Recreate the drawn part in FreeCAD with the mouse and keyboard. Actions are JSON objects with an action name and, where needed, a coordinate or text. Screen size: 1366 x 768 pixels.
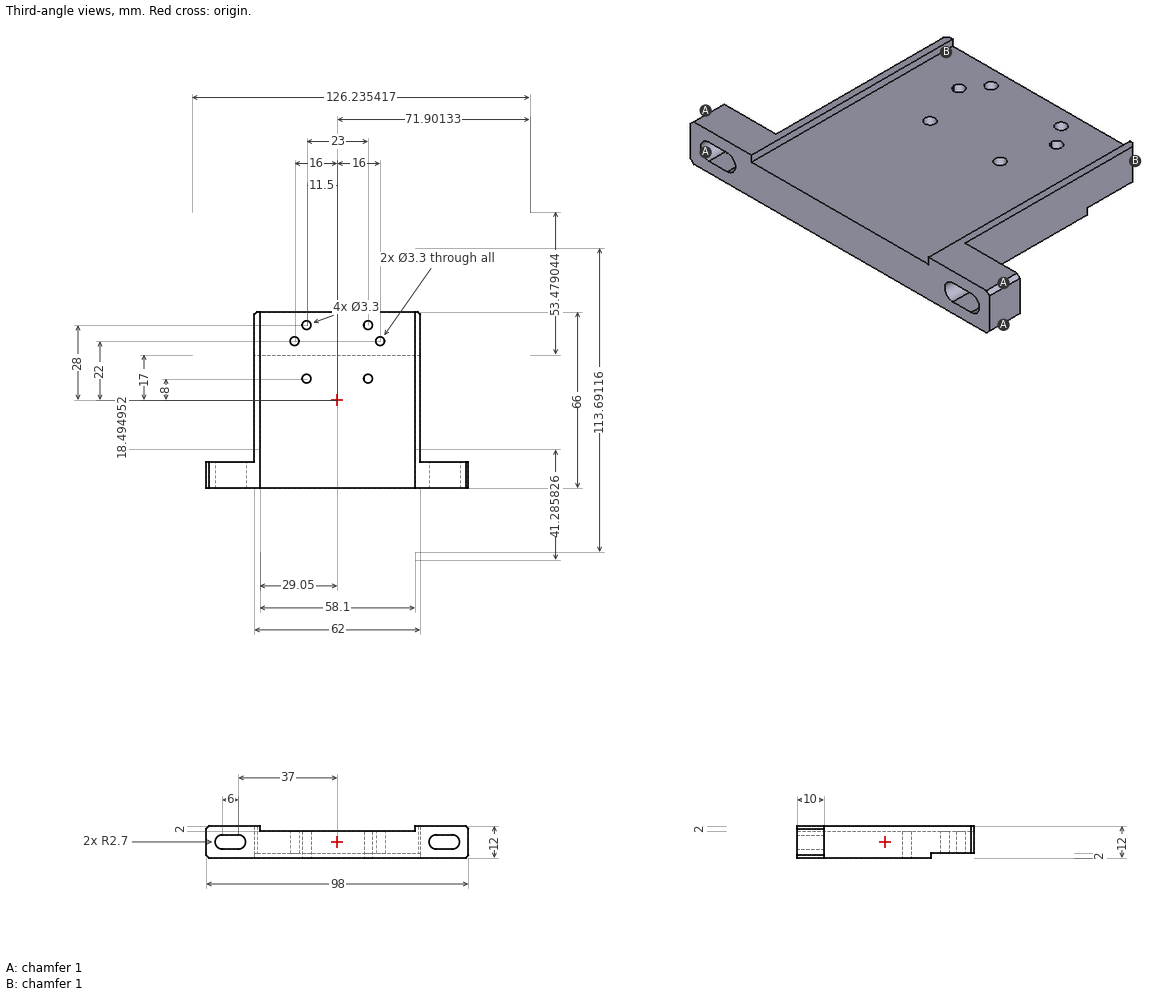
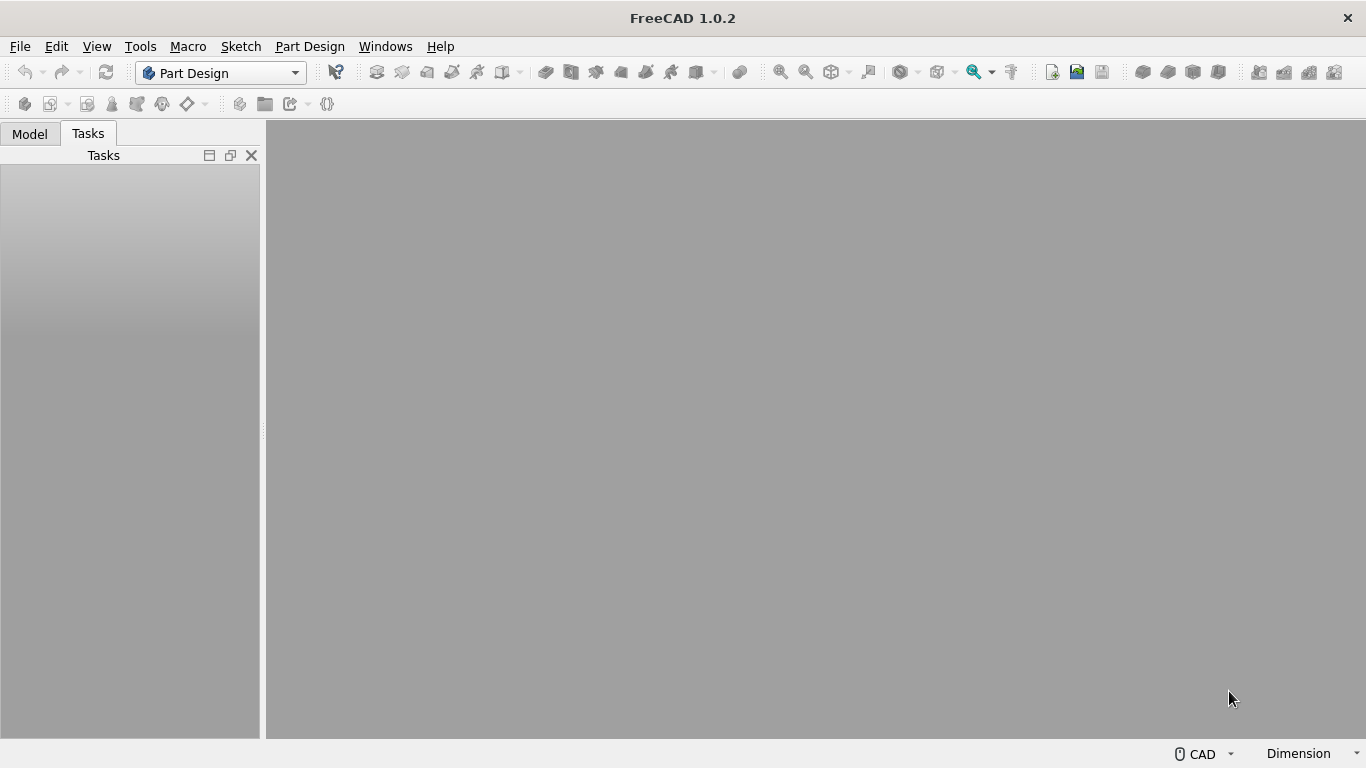
{"action": "left_click", "coordinate": [1052, 72]}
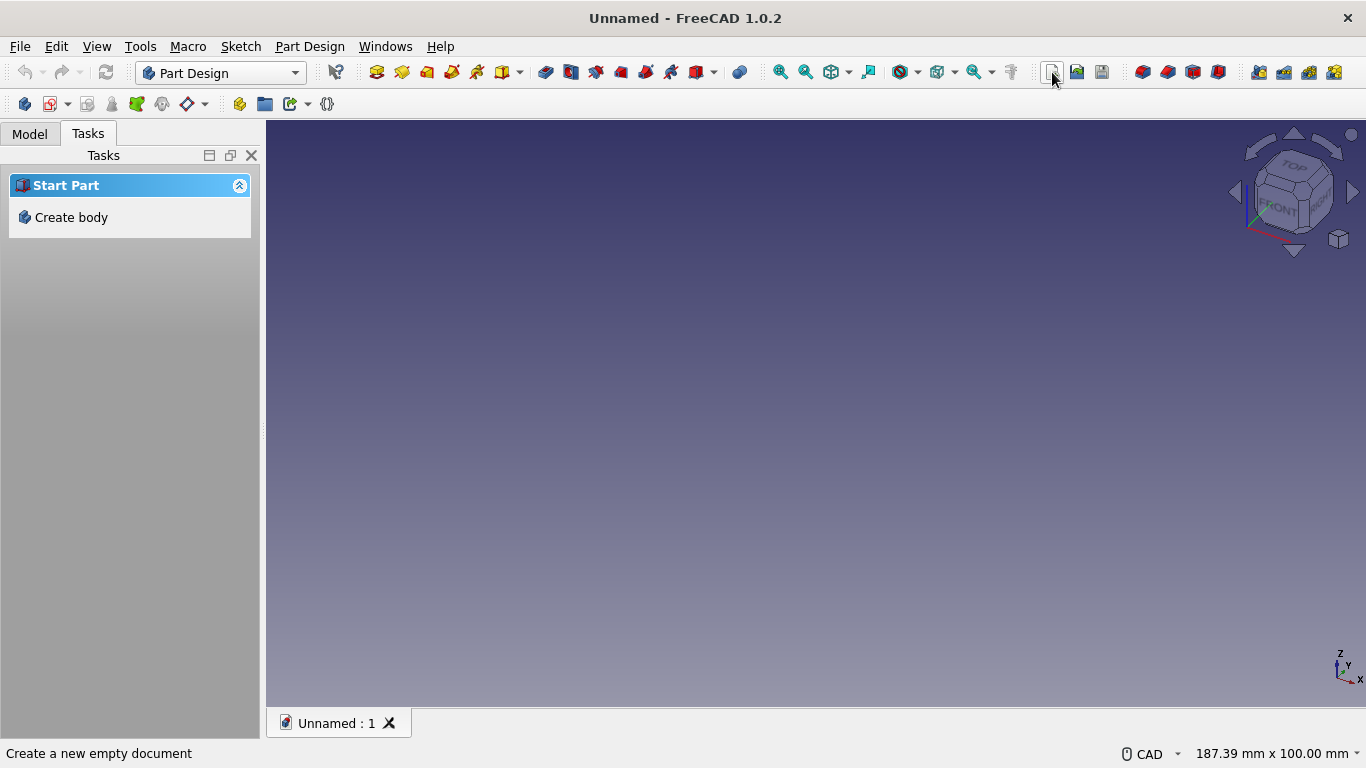
{"action": "left_click", "coordinate": [50, 104]}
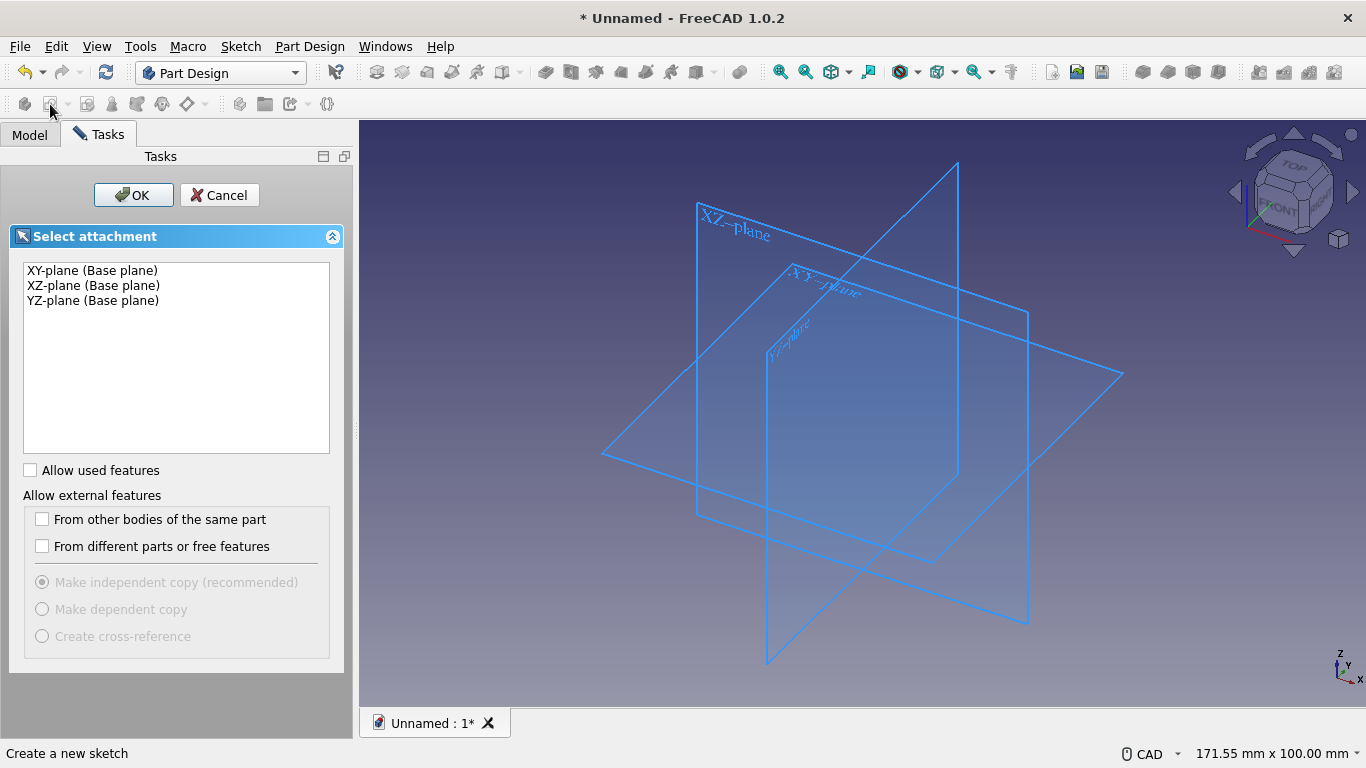
{"action": "left_click", "coordinate": [84, 270]}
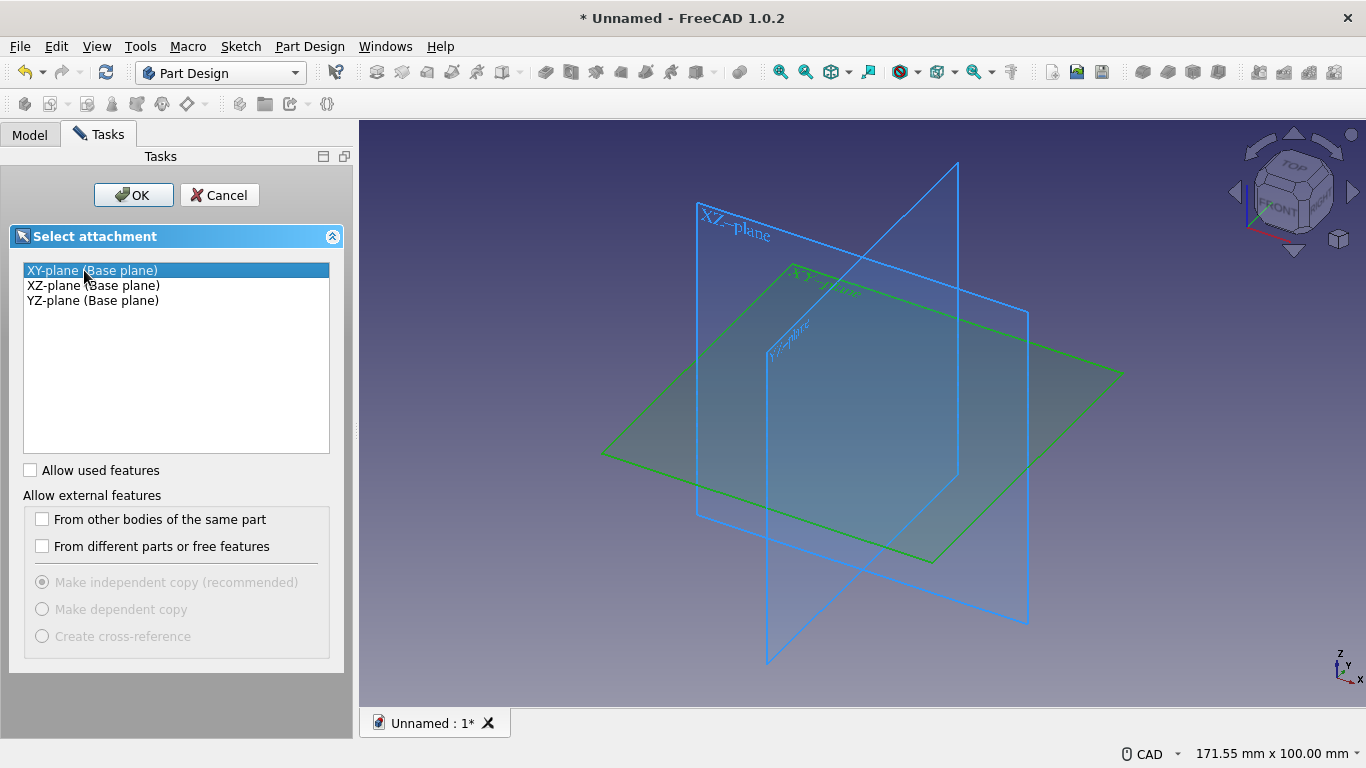
{"action": "left_click", "coordinate": [134, 195]}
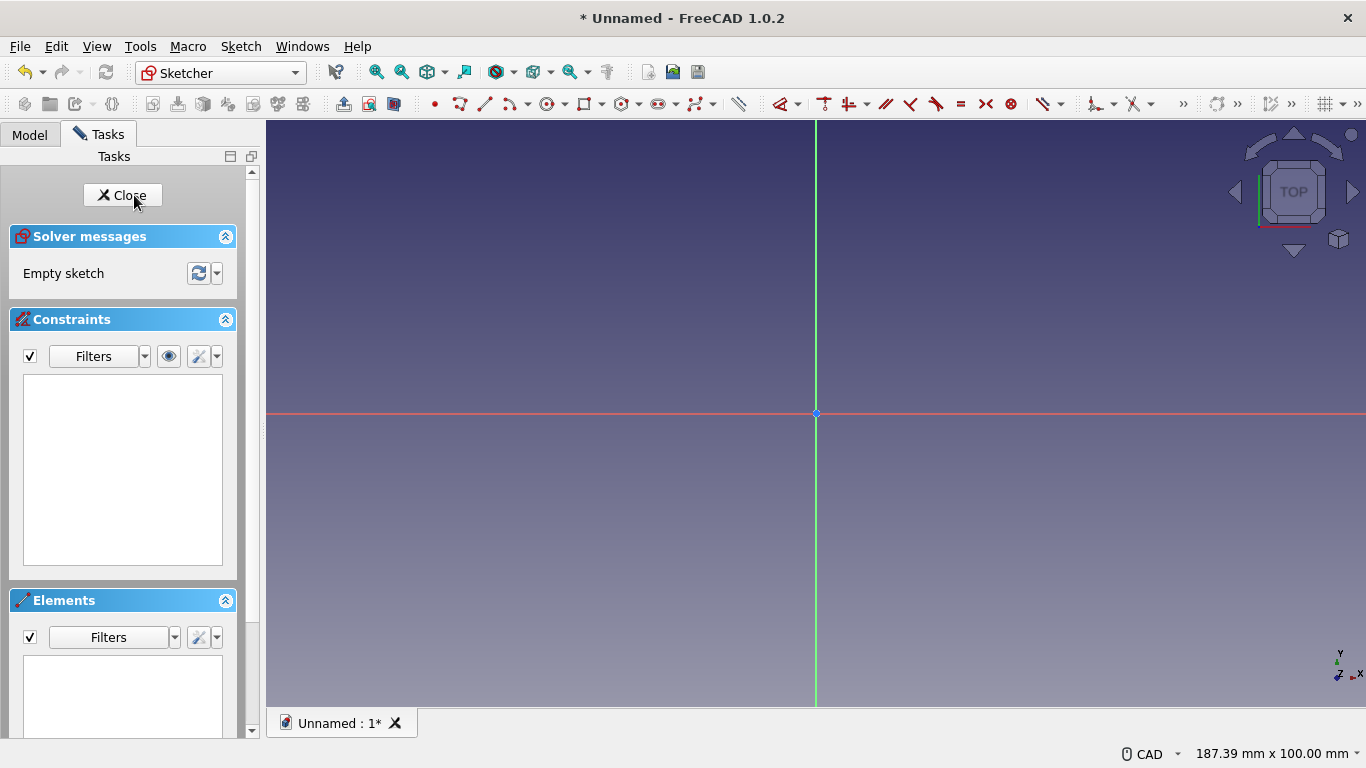
{"action": "left_click", "coordinate": [602, 104]}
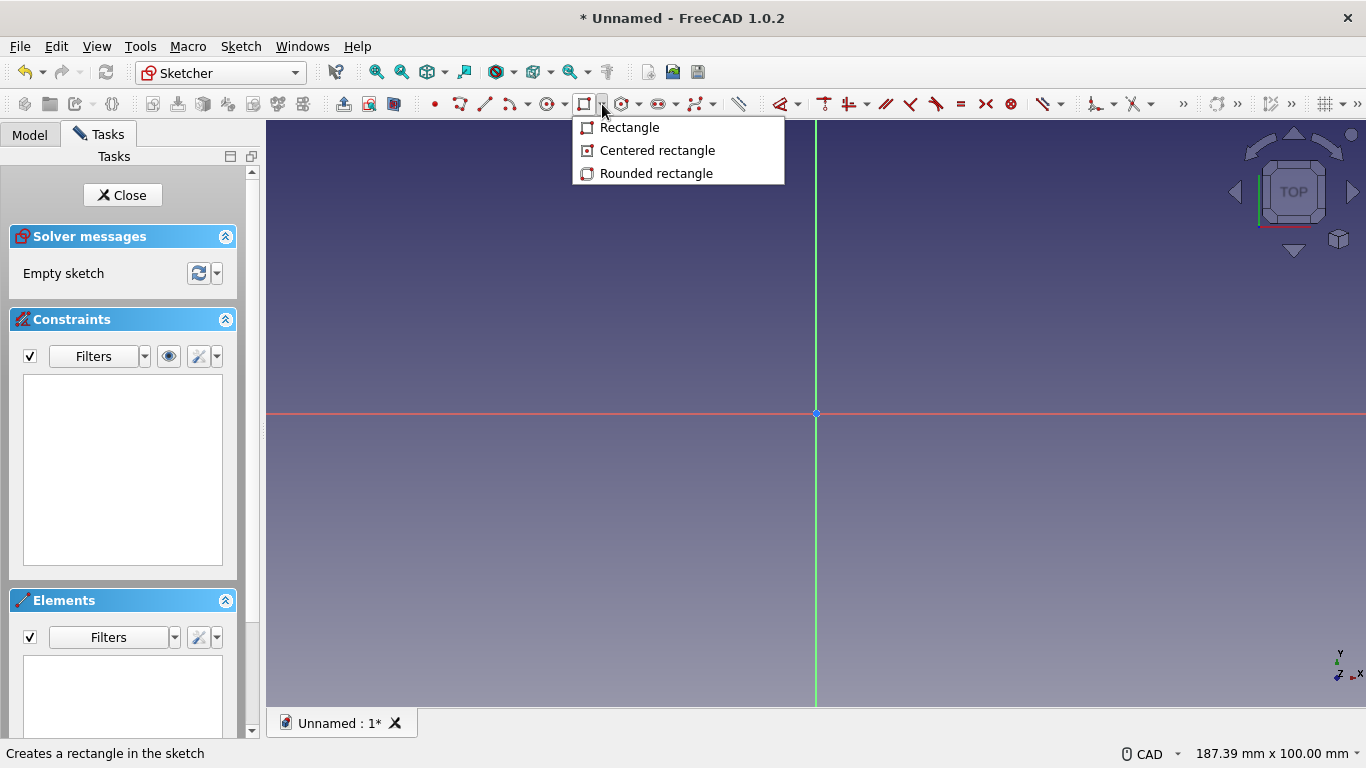
{"action": "left_click", "coordinate": [678, 150]}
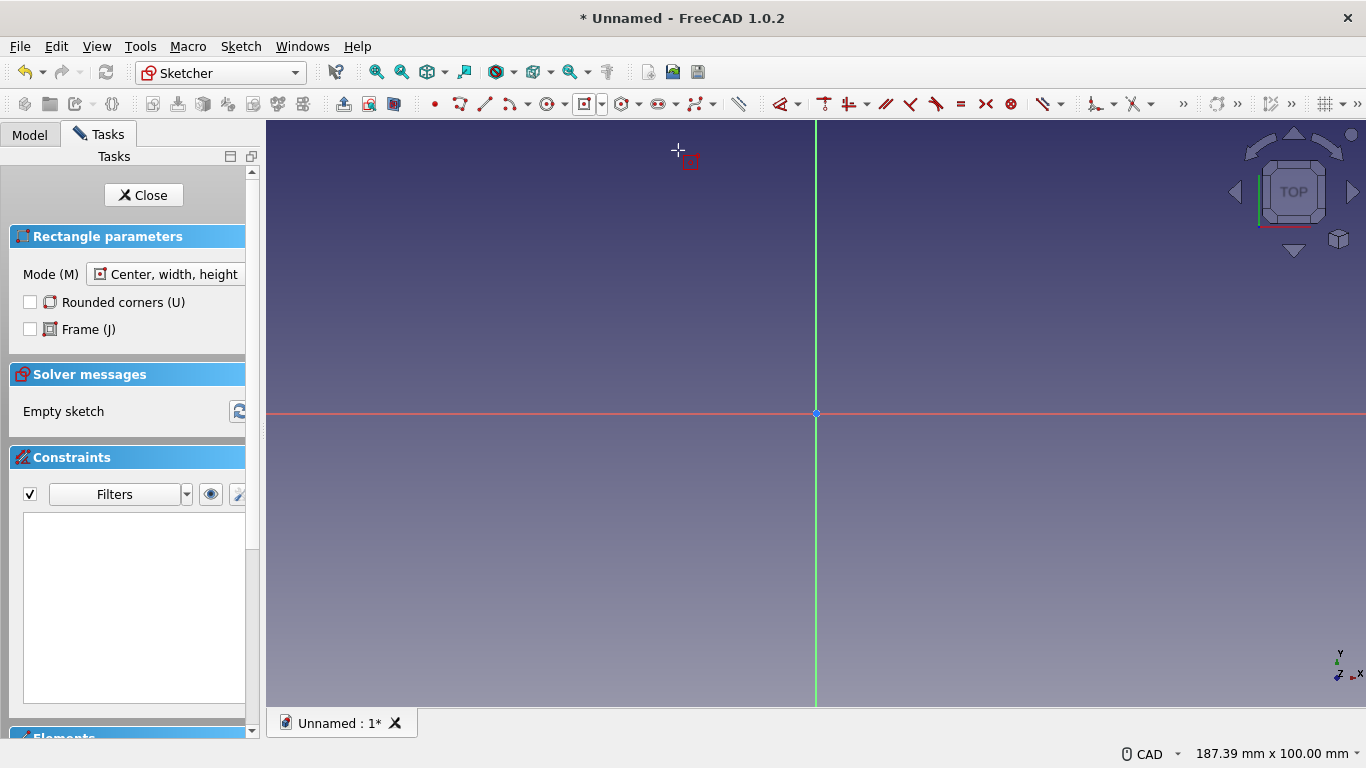
{"action": "left_click", "coordinate": [816, 414]}
{"action": "mouse_move", "coordinate": [998, 220]}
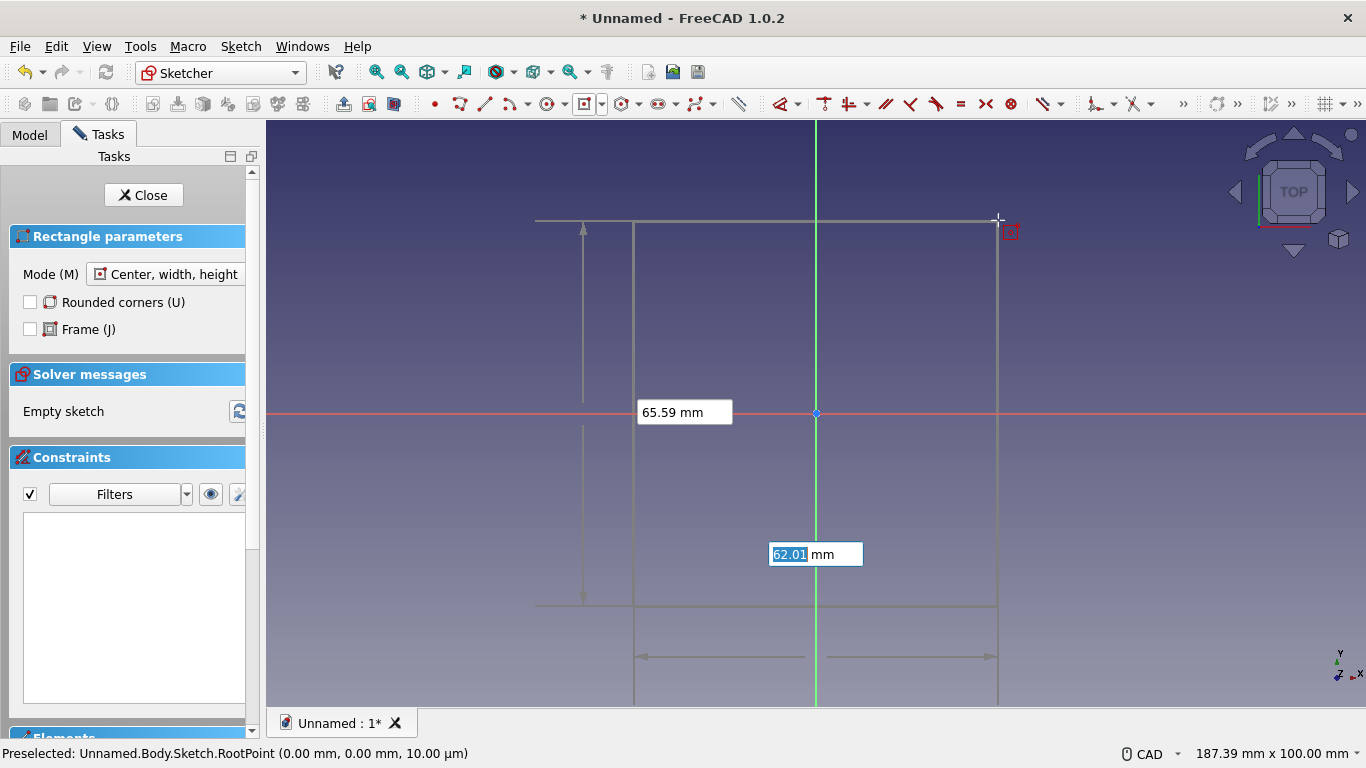
{"action": "type", "text": "62"}
{"action": "key", "text": "Tab"}
{"action": "type", "text": "66"}
{"action": "key", "text": "Return"}
{"action": "key", "text": "Escape"}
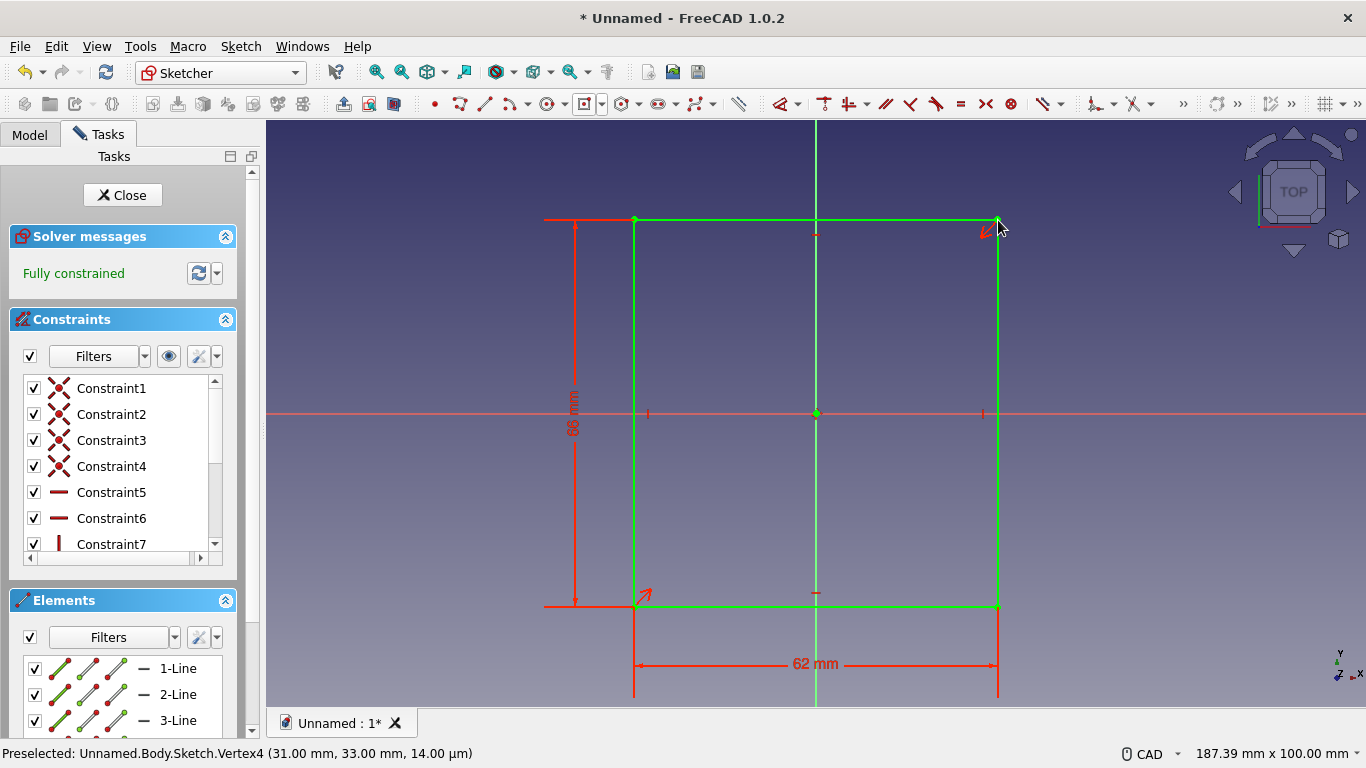
{"action": "left_click", "coordinate": [123, 195]}